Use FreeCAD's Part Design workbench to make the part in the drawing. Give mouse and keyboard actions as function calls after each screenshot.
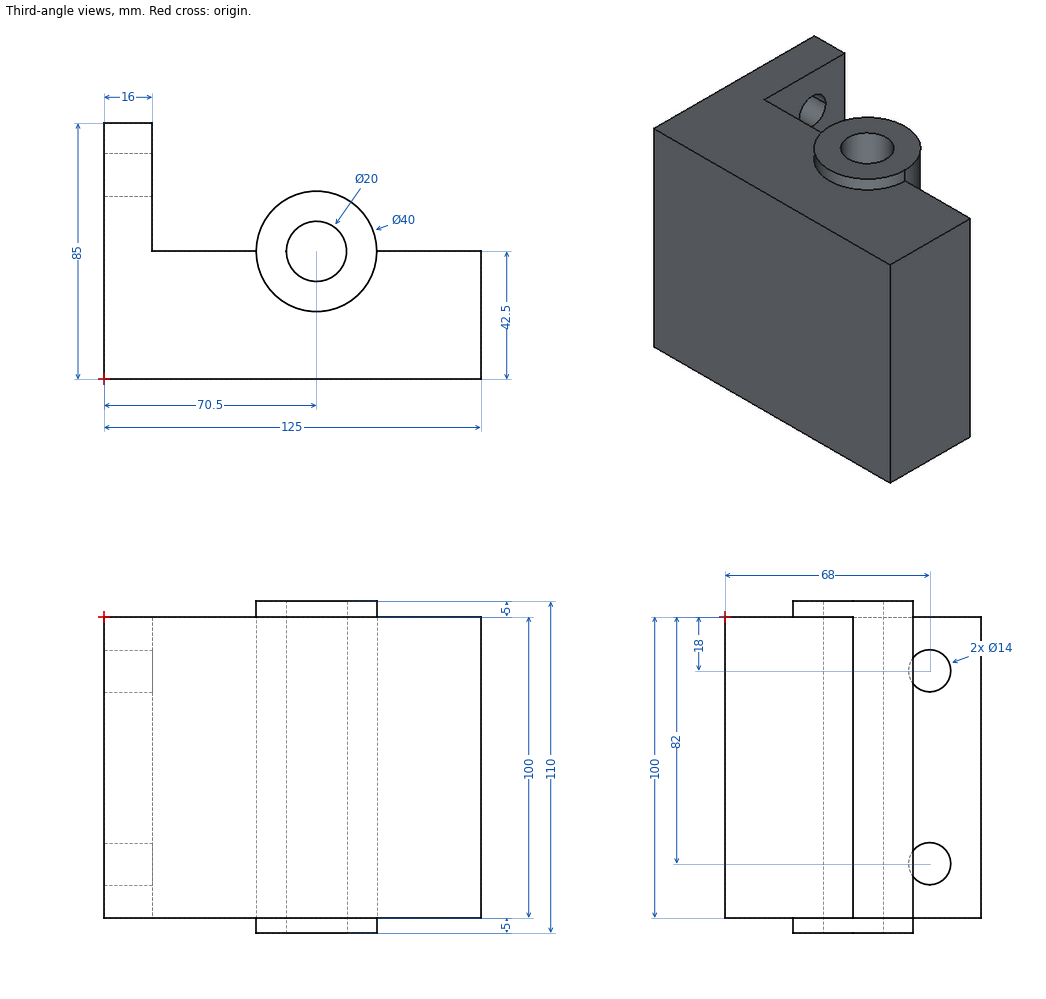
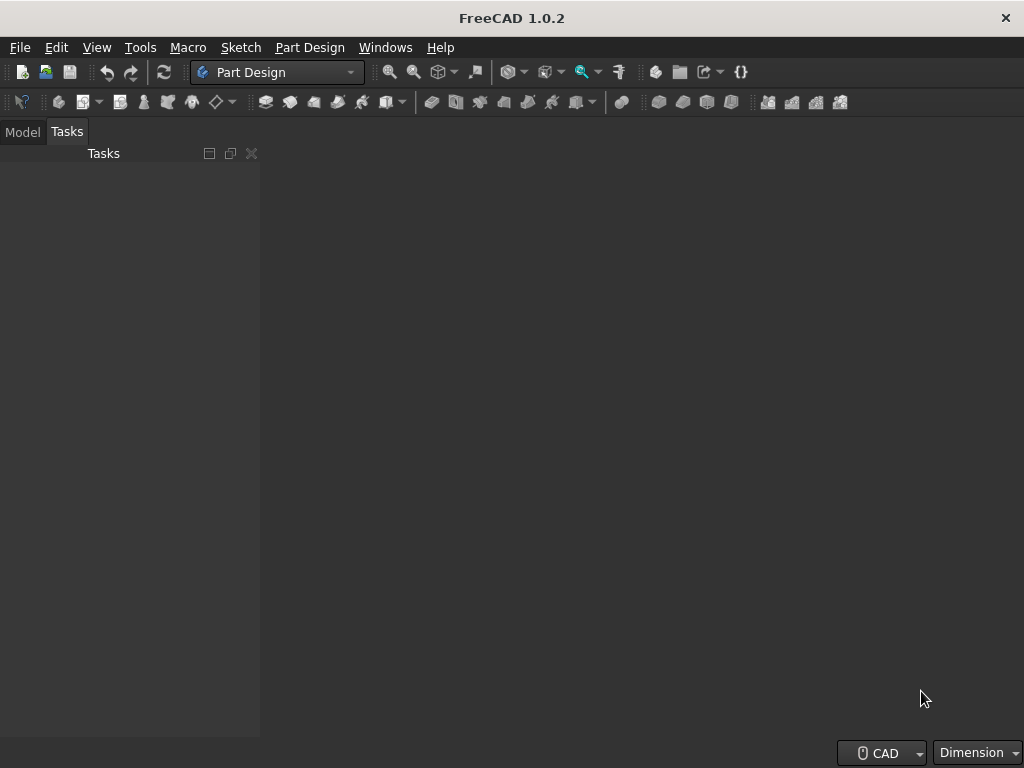
click(22, 72)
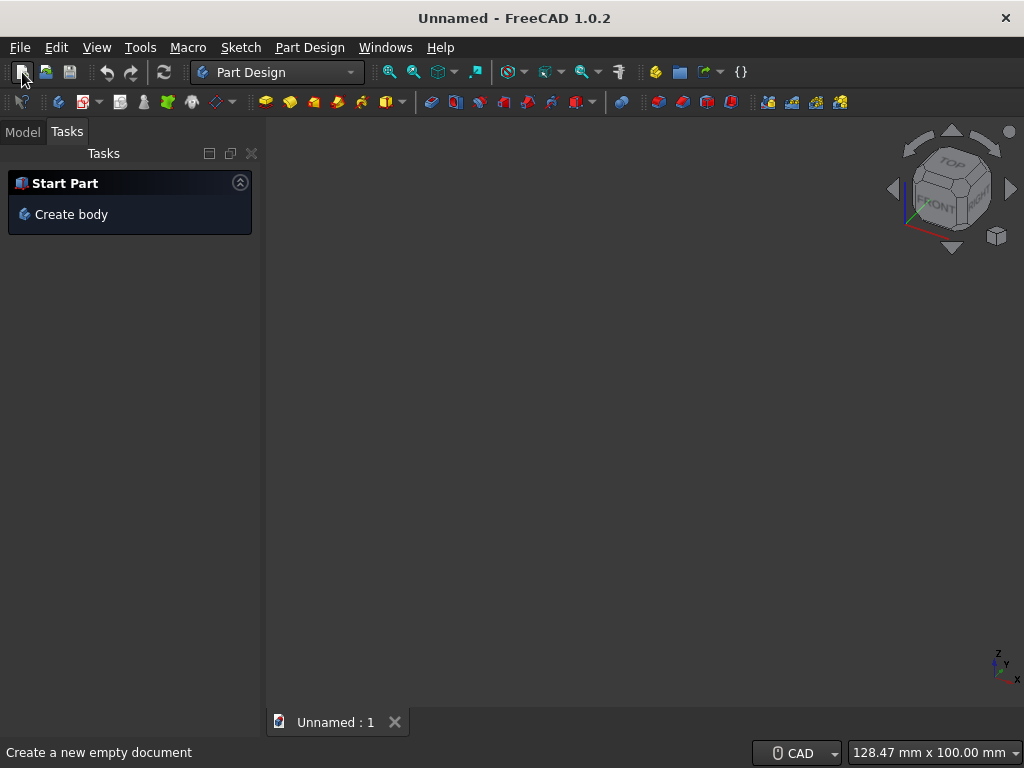
click(84, 102)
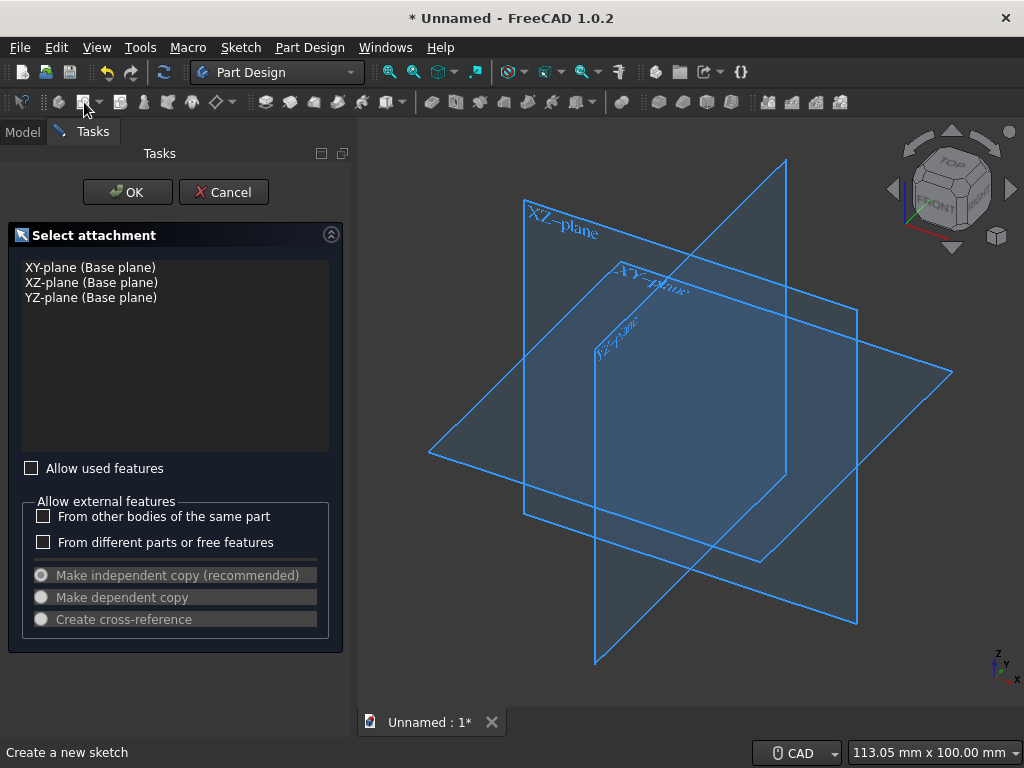
click(82, 268)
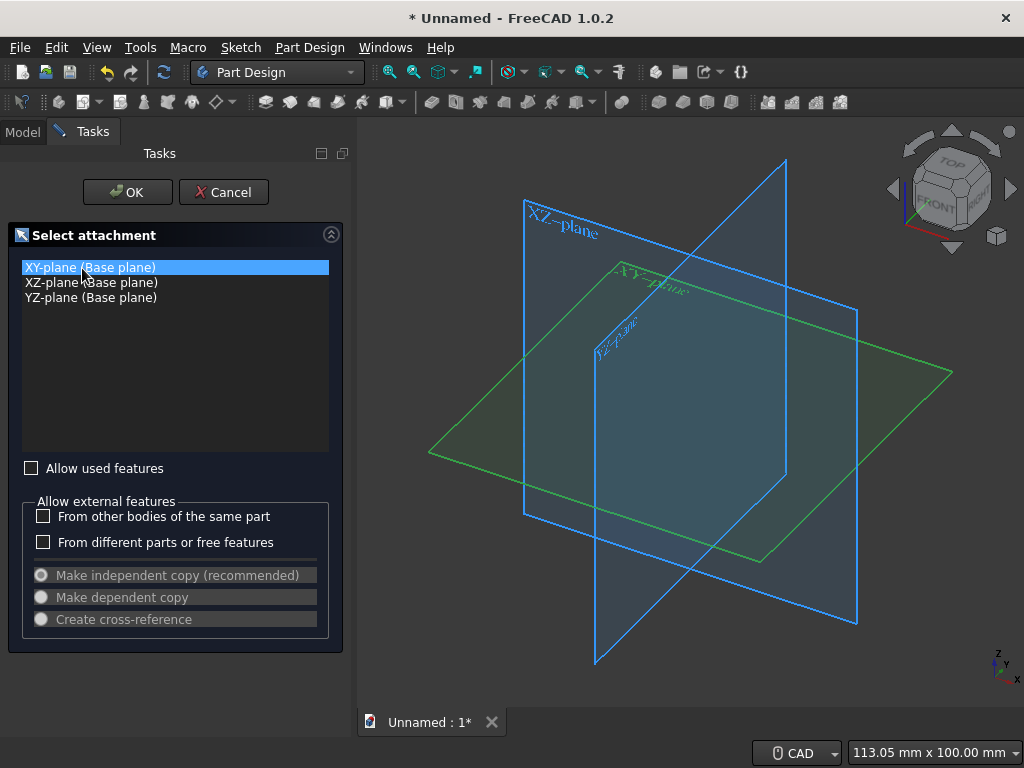
click(128, 192)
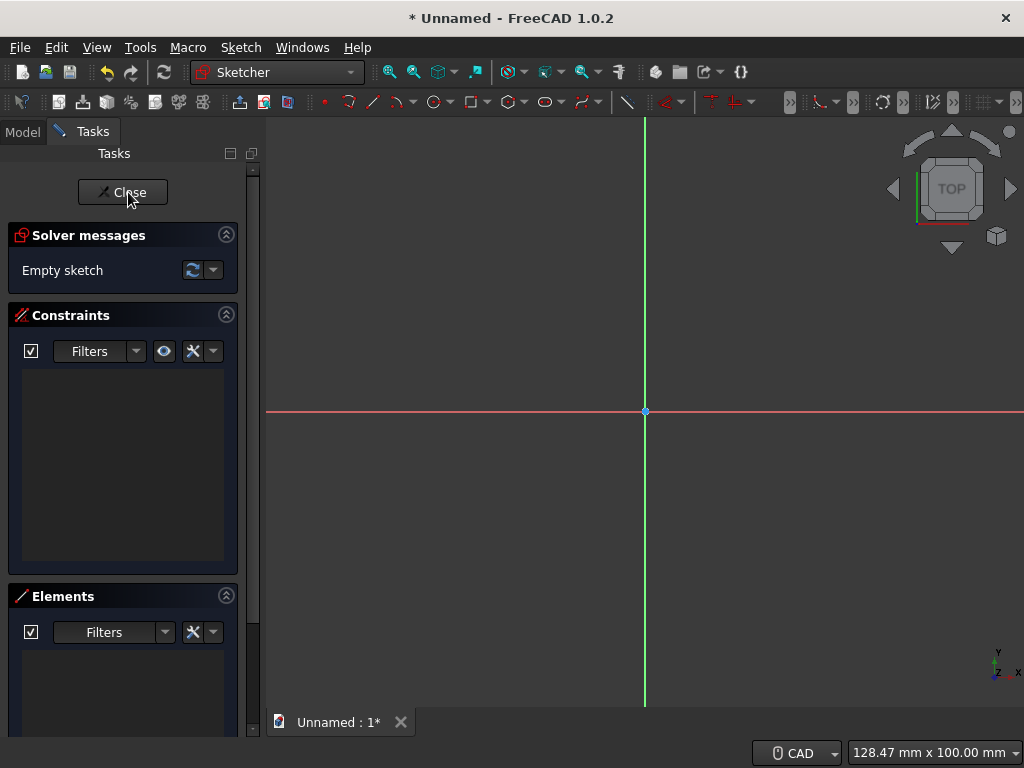
scroll(294, 617, down, 4)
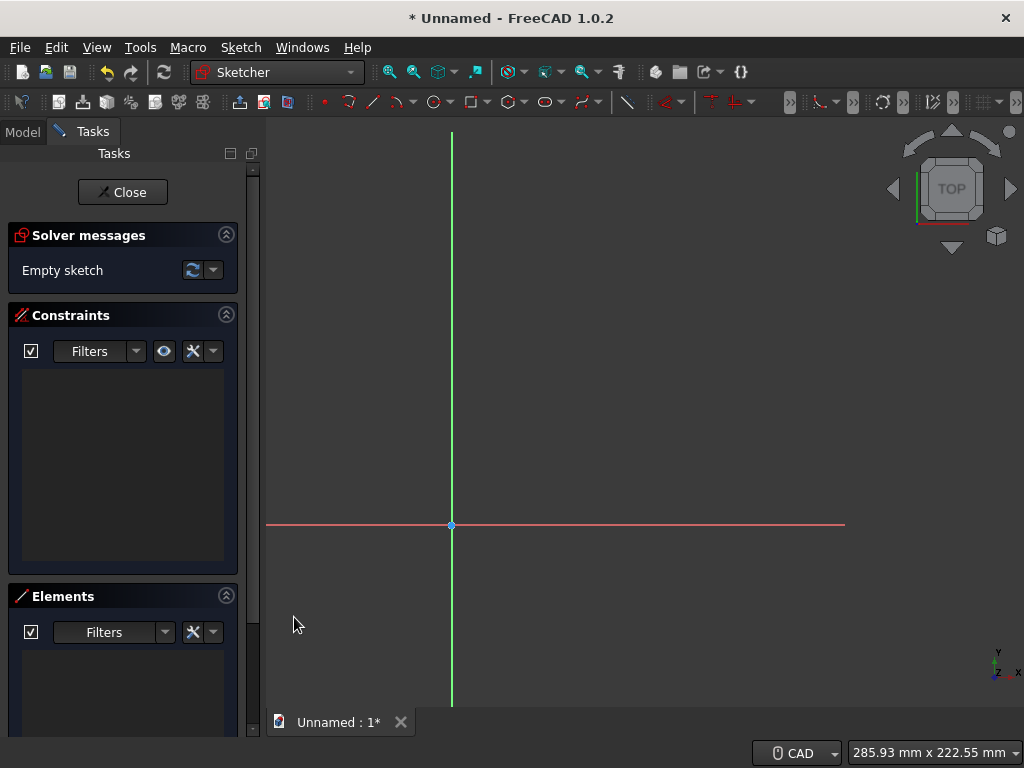
click(350, 102)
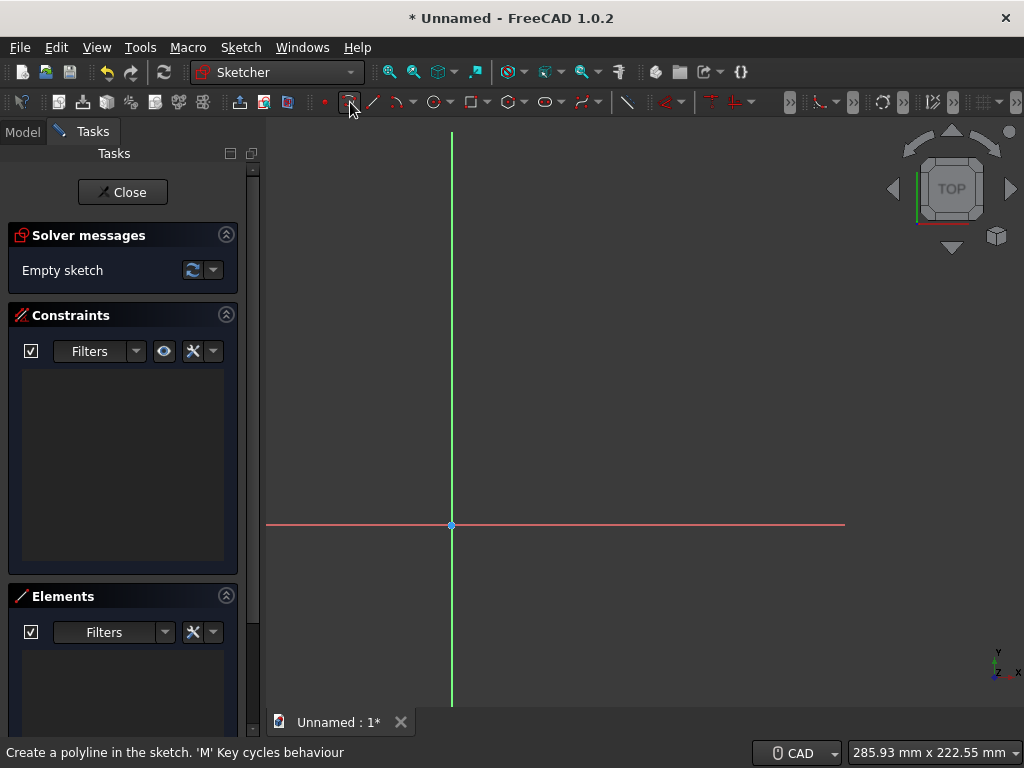
click(452, 525)
click(783, 516)
click(783, 413)
click(494, 413)
click(494, 300)
click(461, 300)
click(452, 525)
key(Escape)
key(Escape)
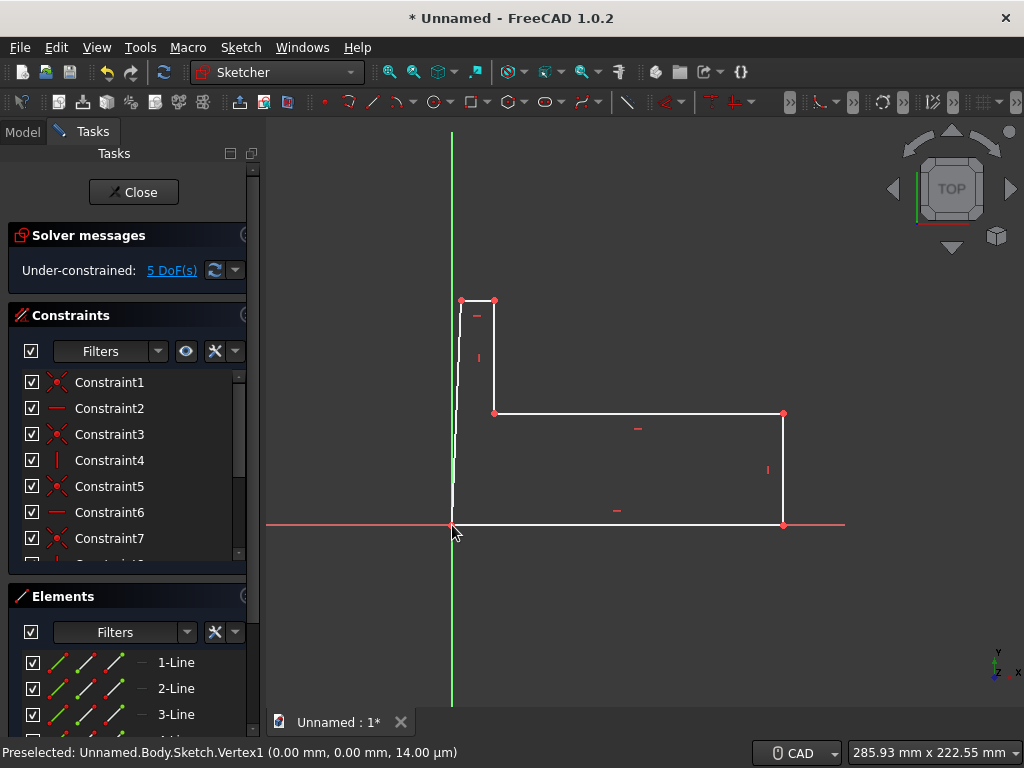
click(455, 458)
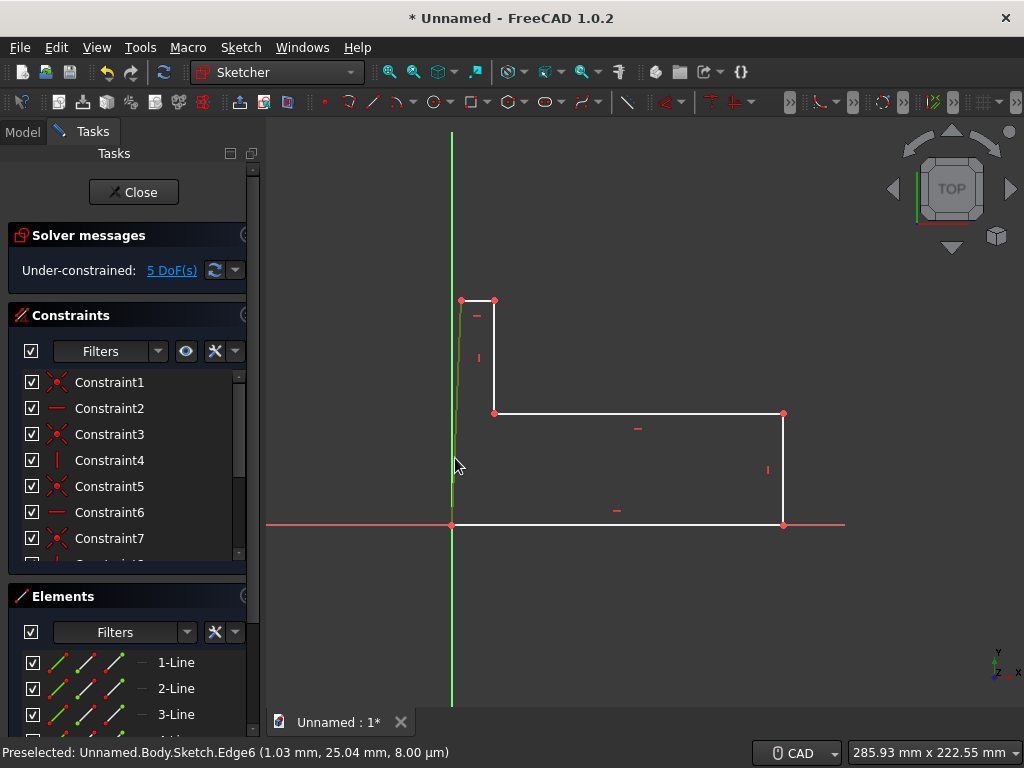
click(754, 102)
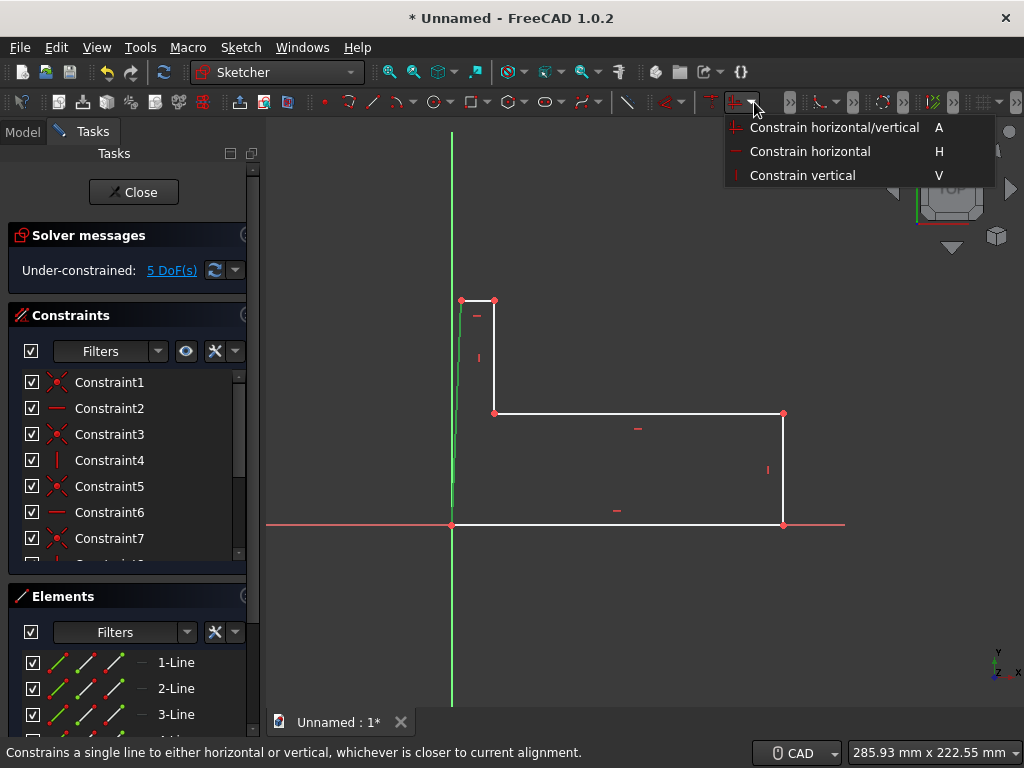
click(860, 175)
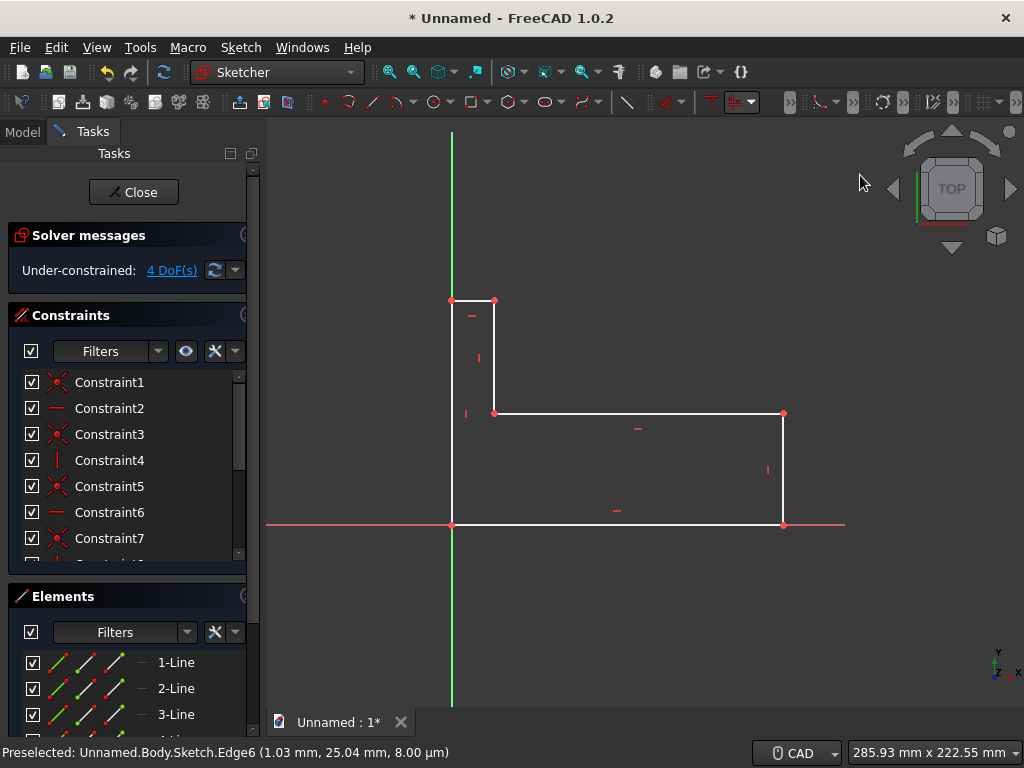
key(d)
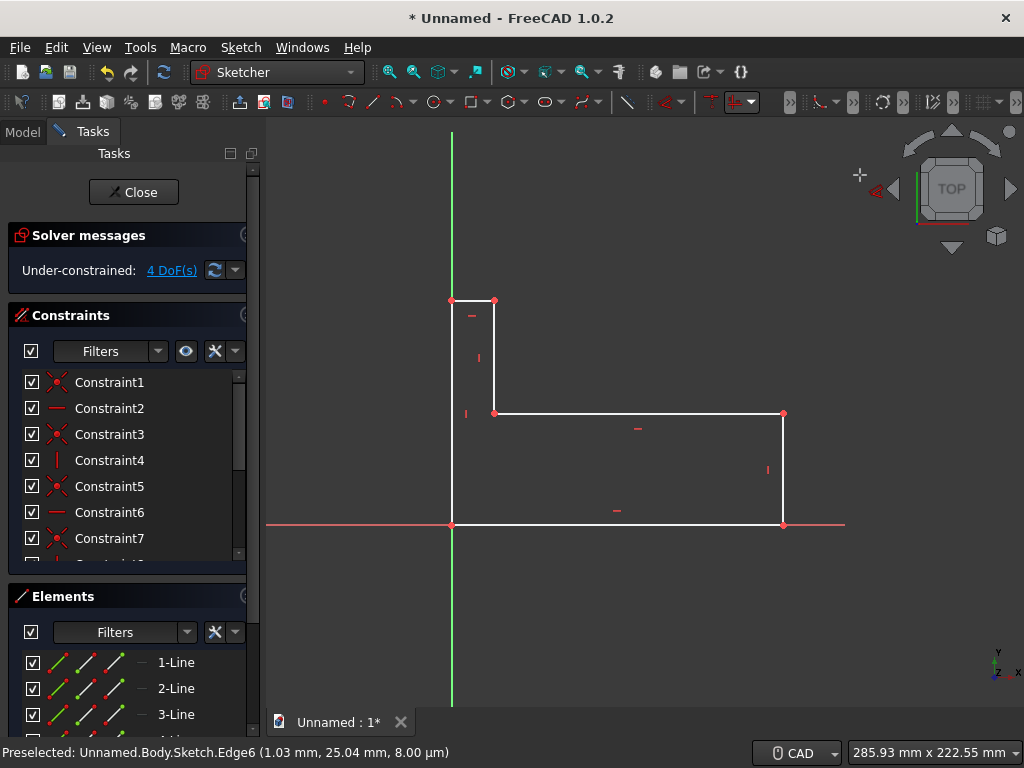
click(481, 301)
click(473, 267)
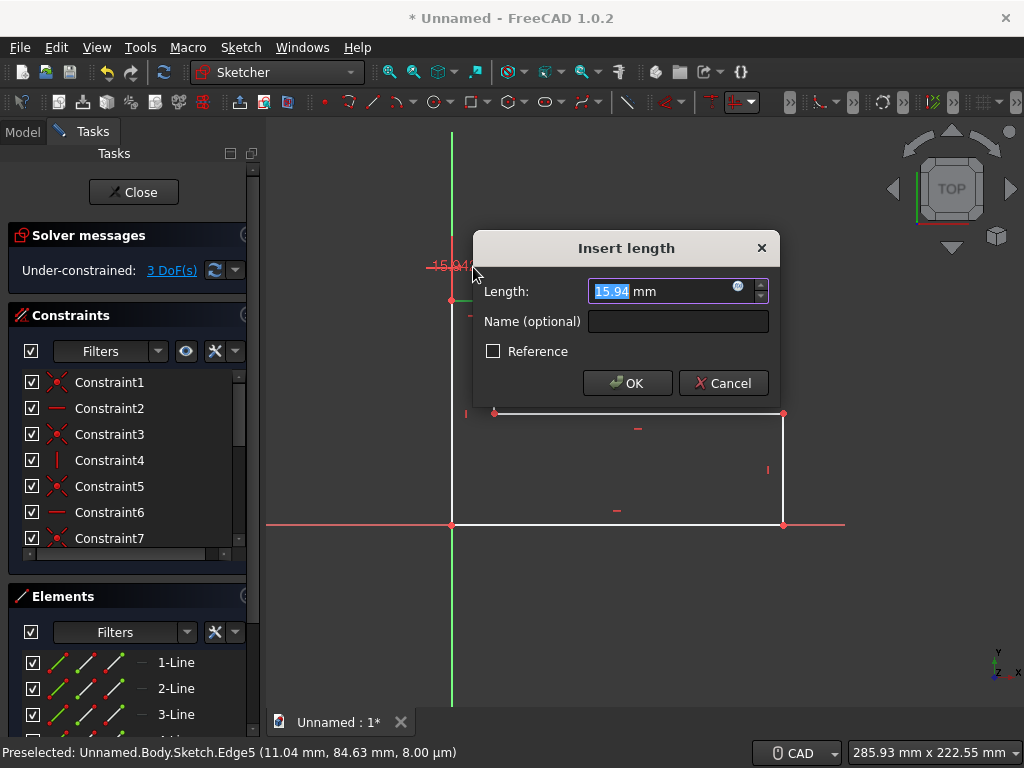
text(16)
key(Return)